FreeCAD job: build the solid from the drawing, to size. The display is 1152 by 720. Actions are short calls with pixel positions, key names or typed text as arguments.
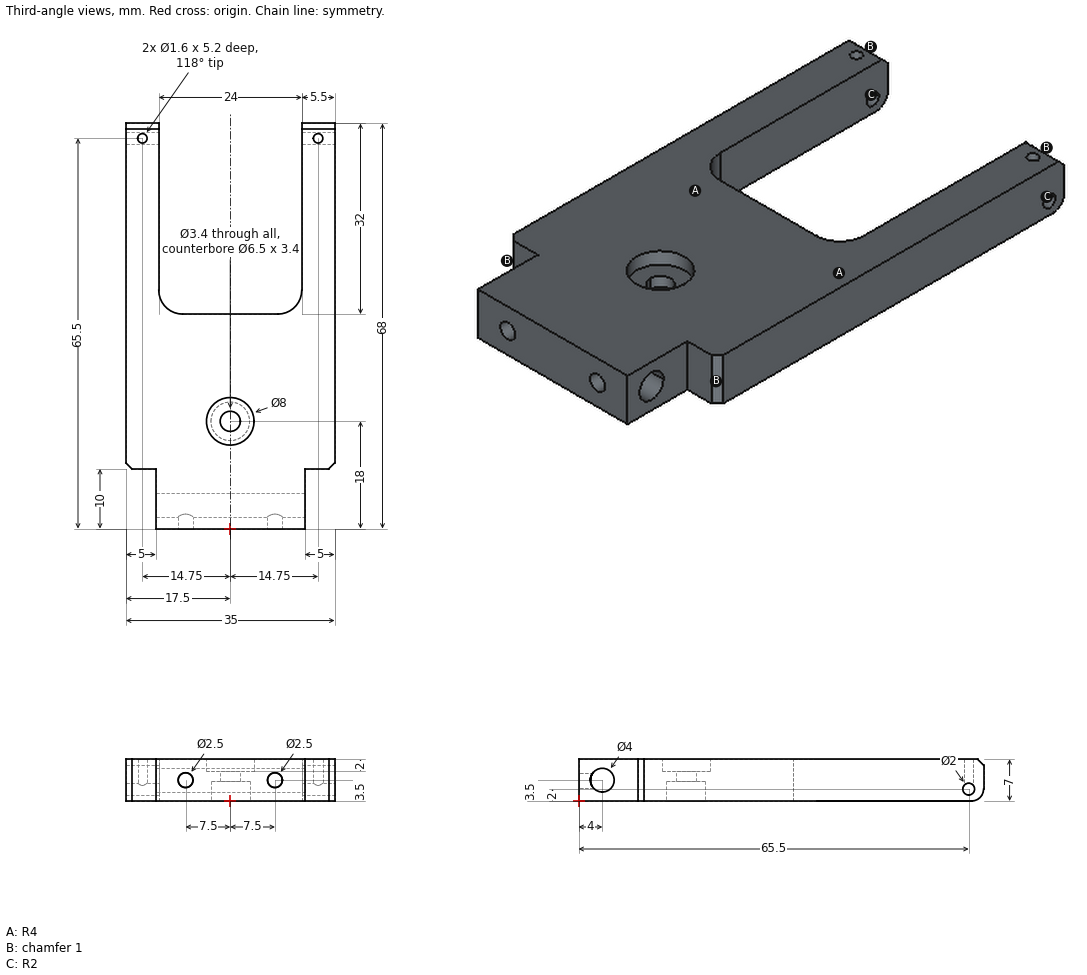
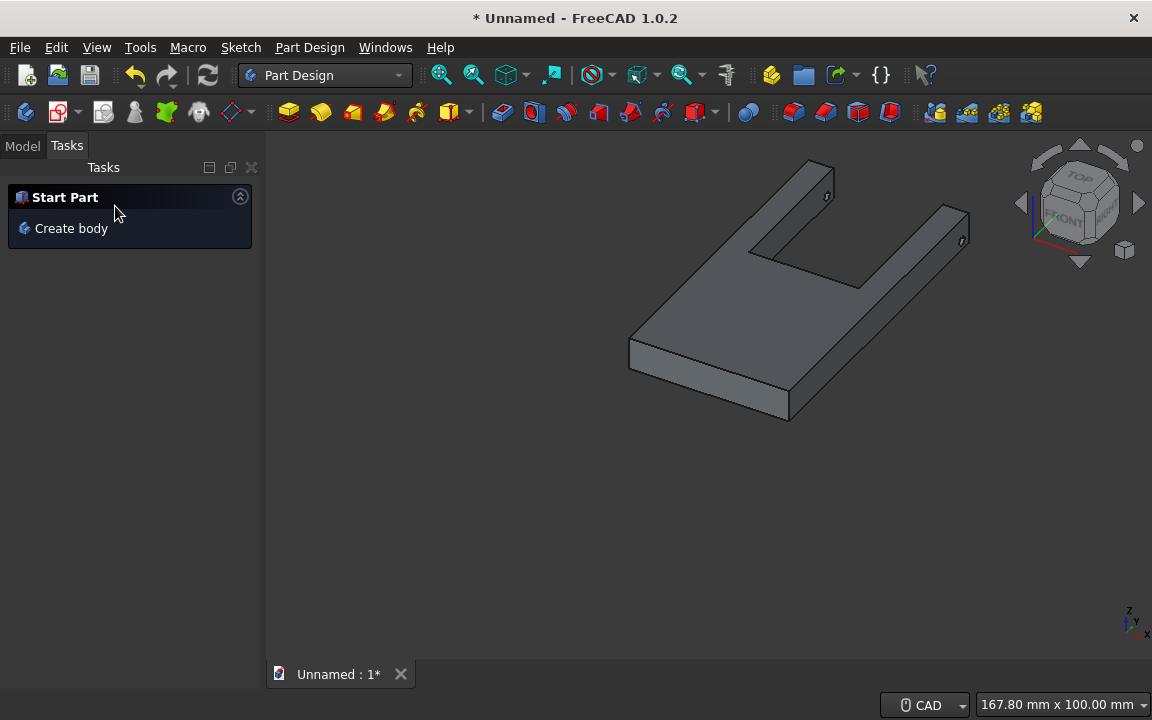
click(747, 326)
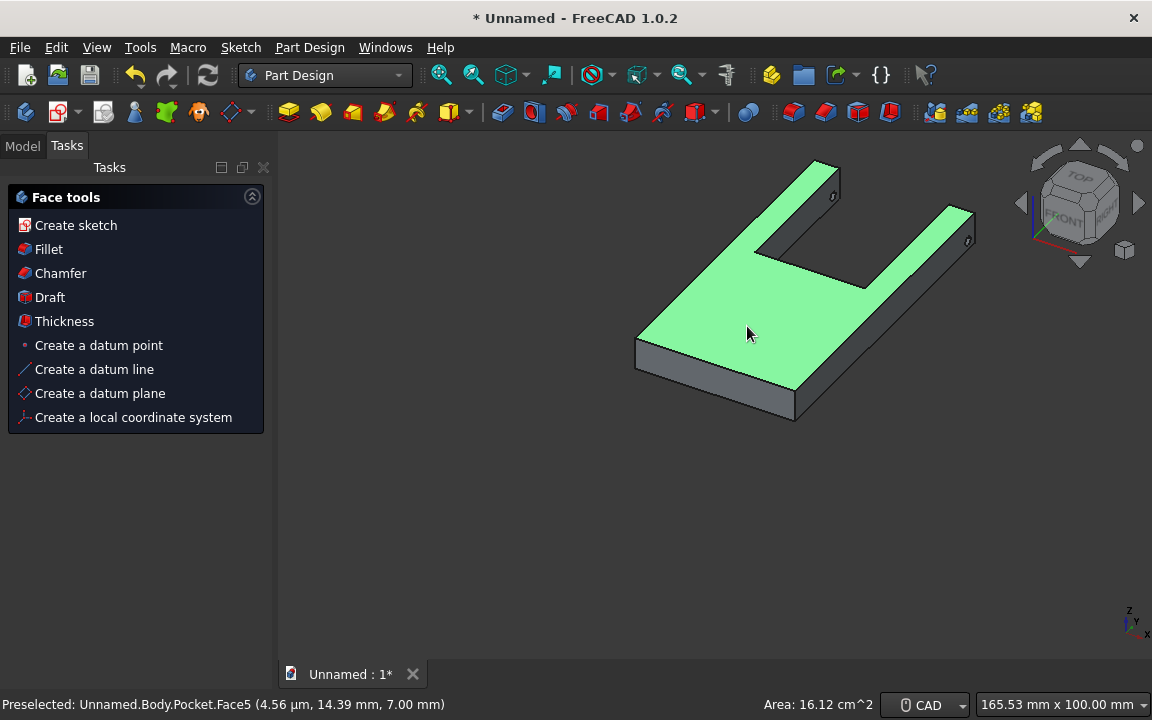
click(58, 112)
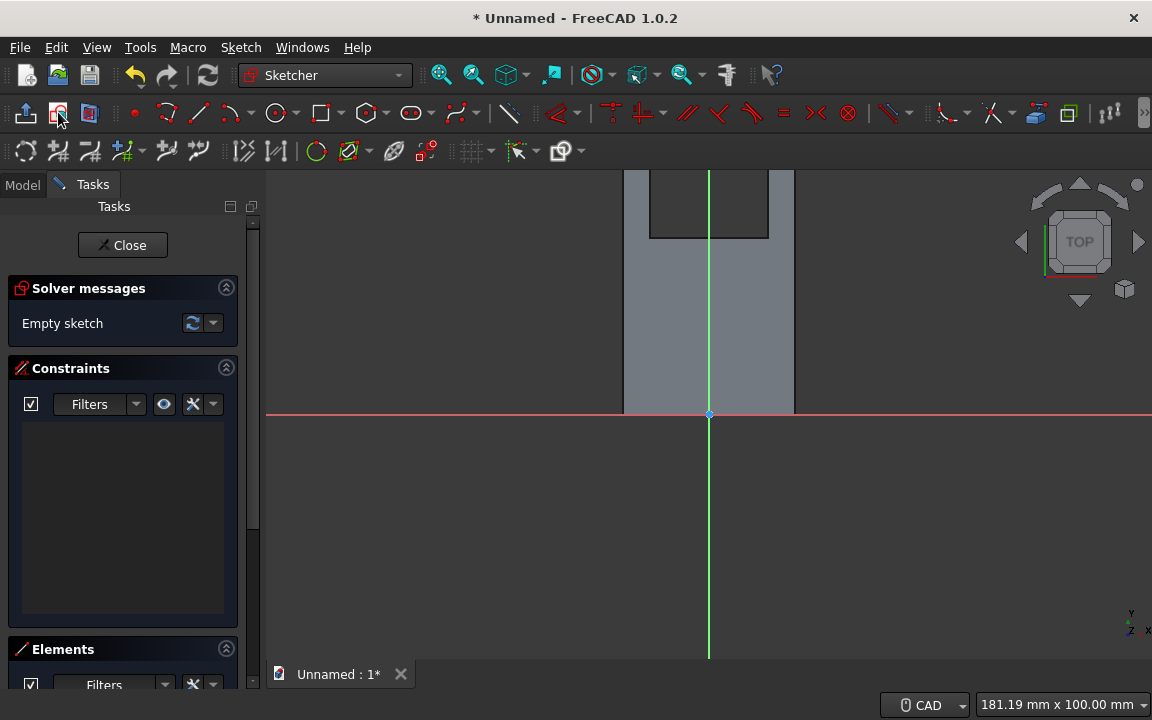
scroll(749, 376, up, 5)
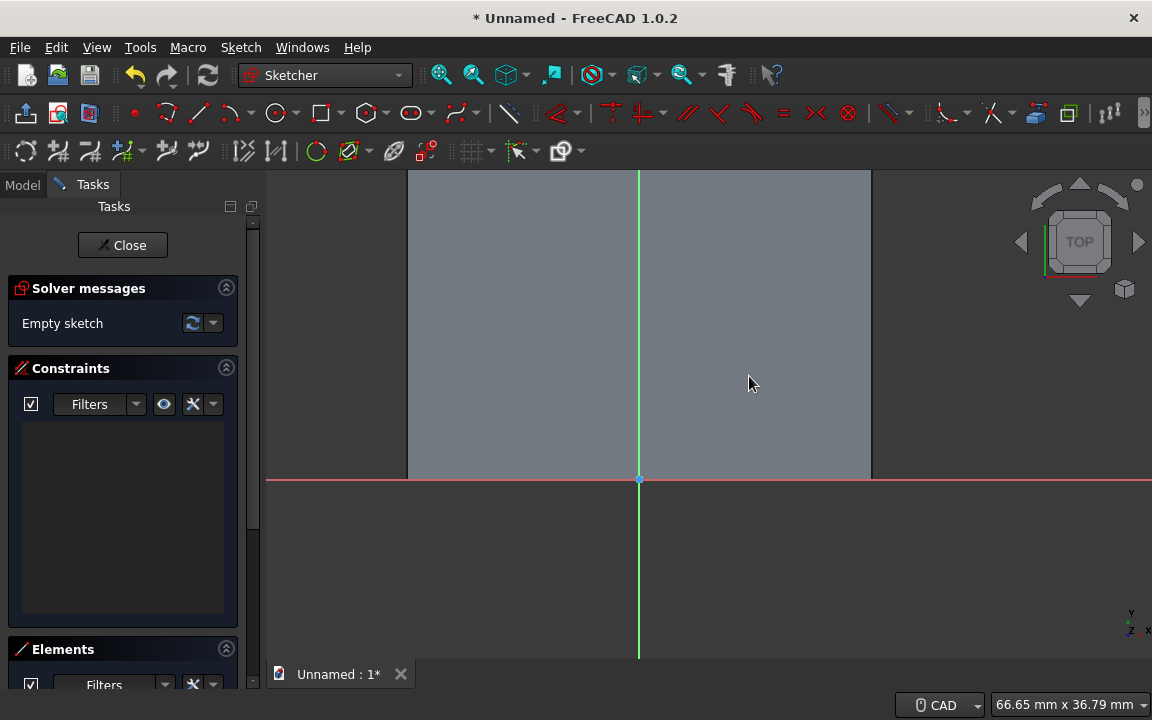
key(g)
key(r)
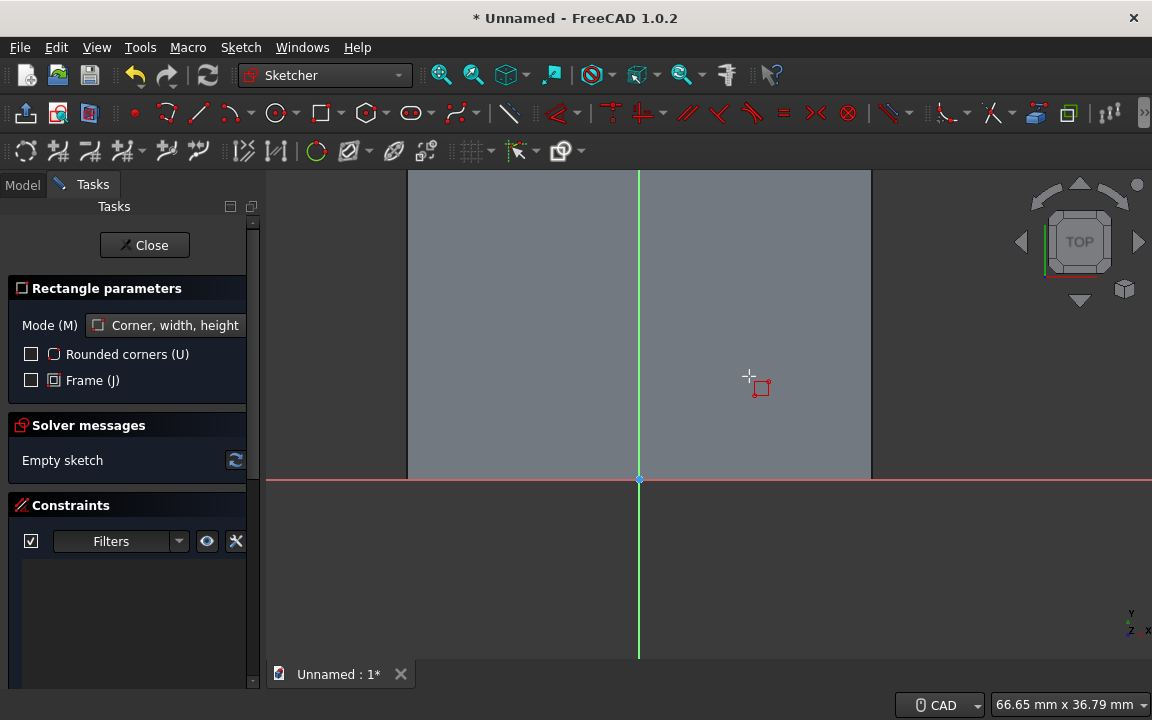
click(407, 347)
click(473, 480)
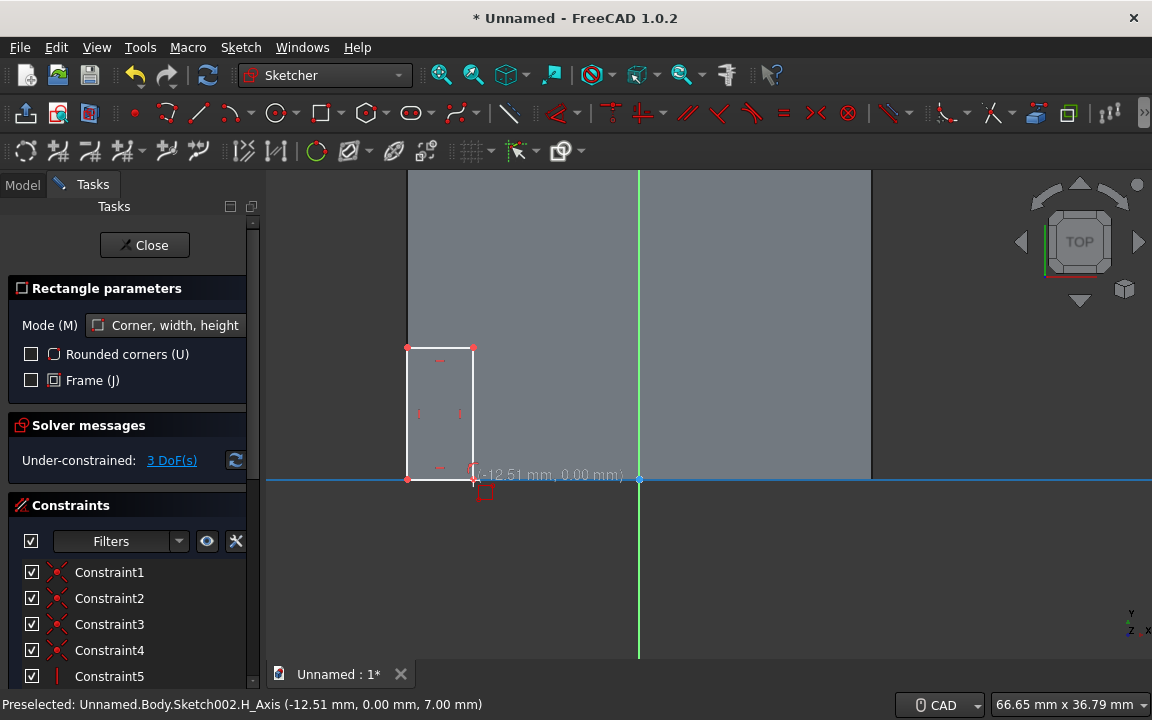
click(805, 347)
click(872, 480)
key(Escape)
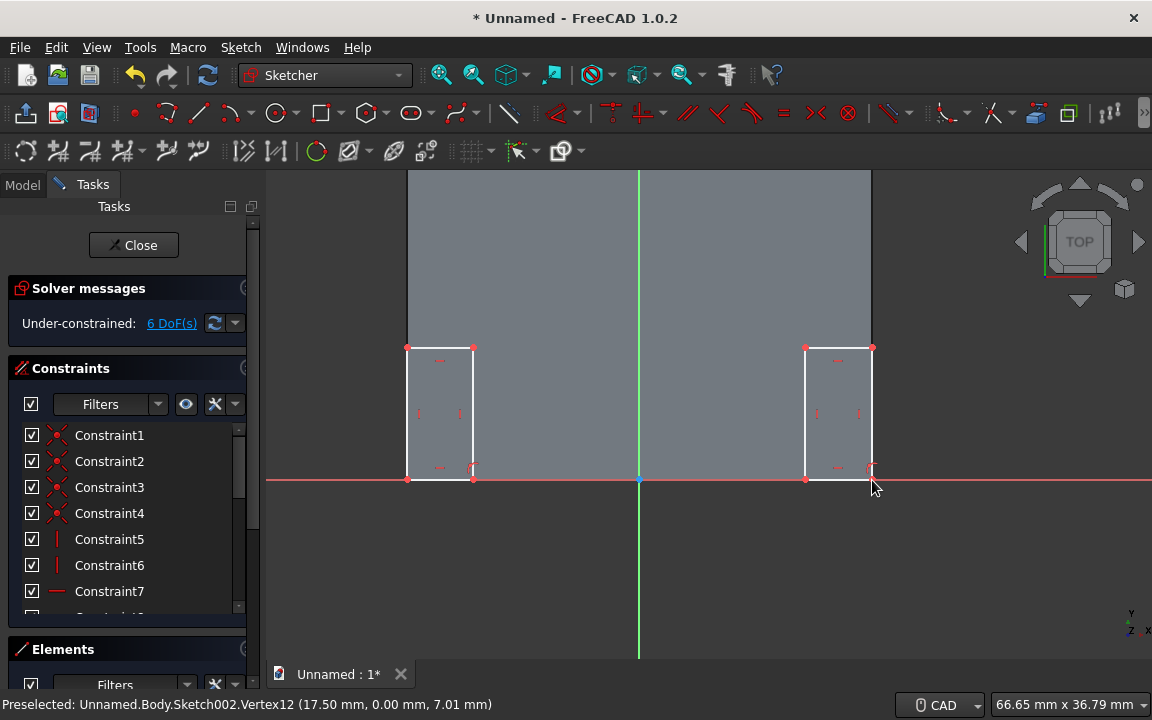
click(473, 348)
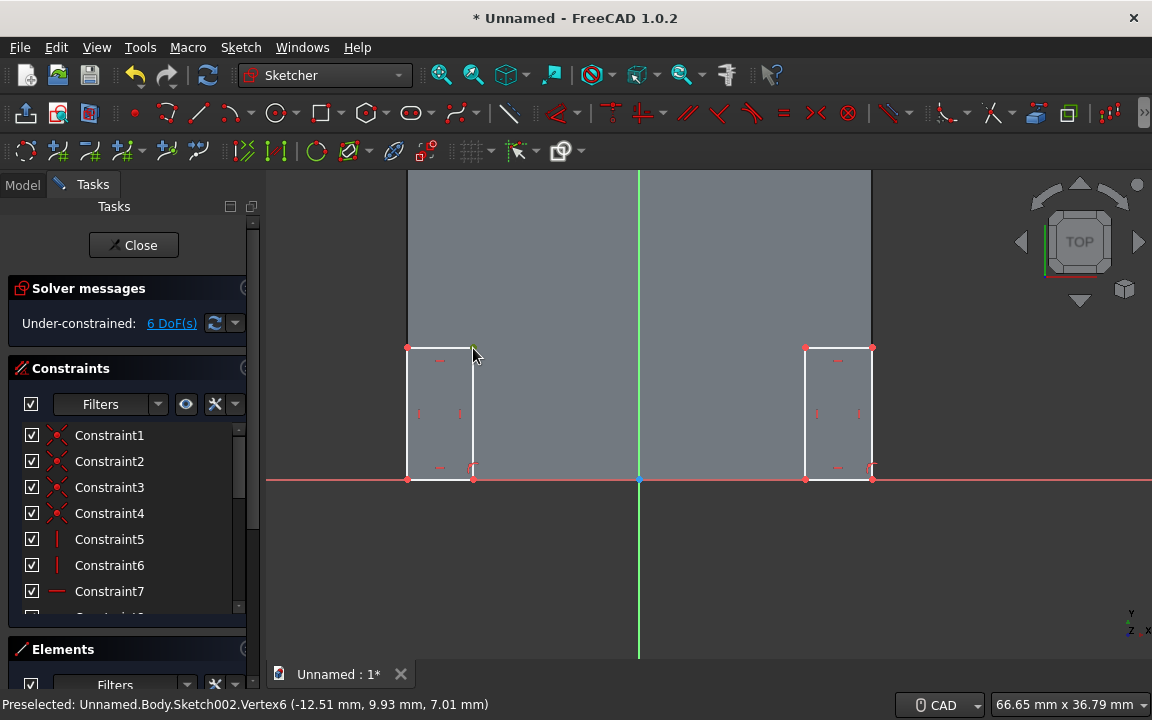
click(805, 348)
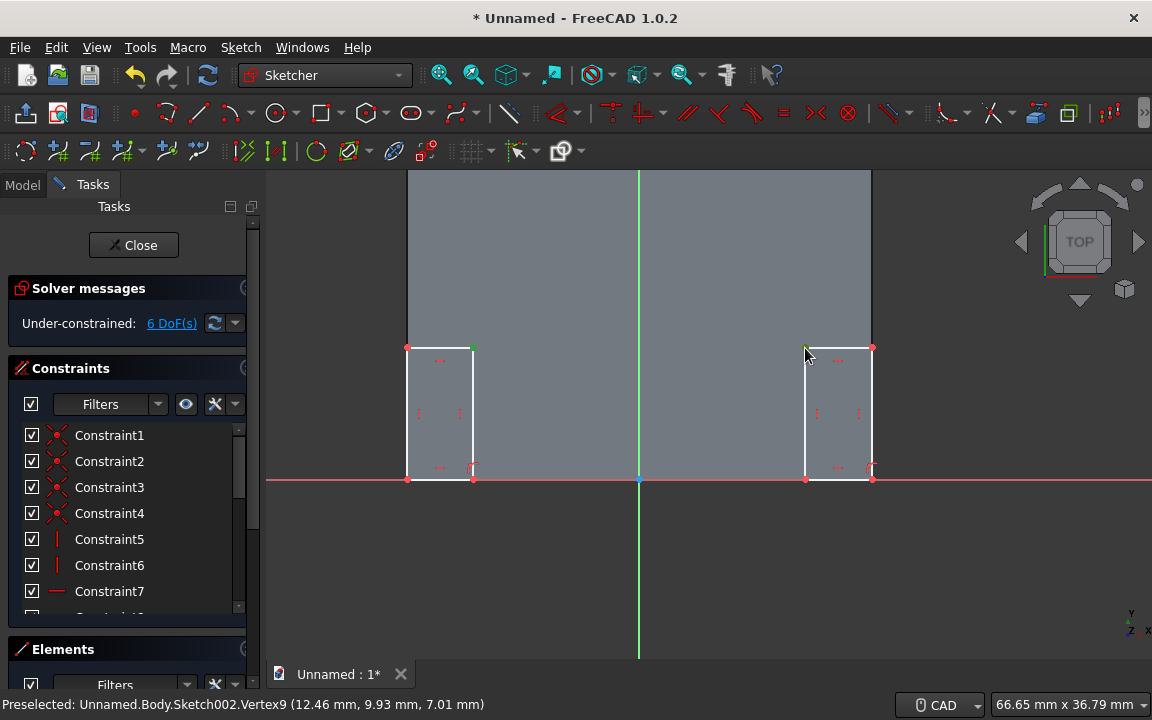
click(639, 600)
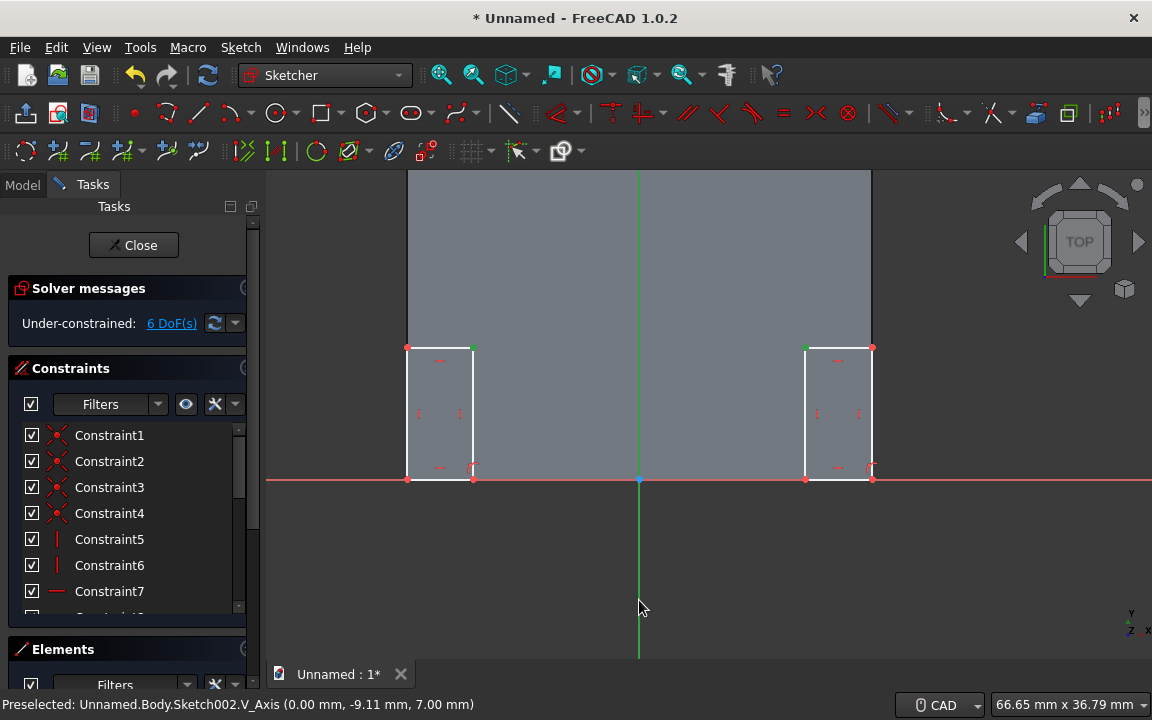
key(s)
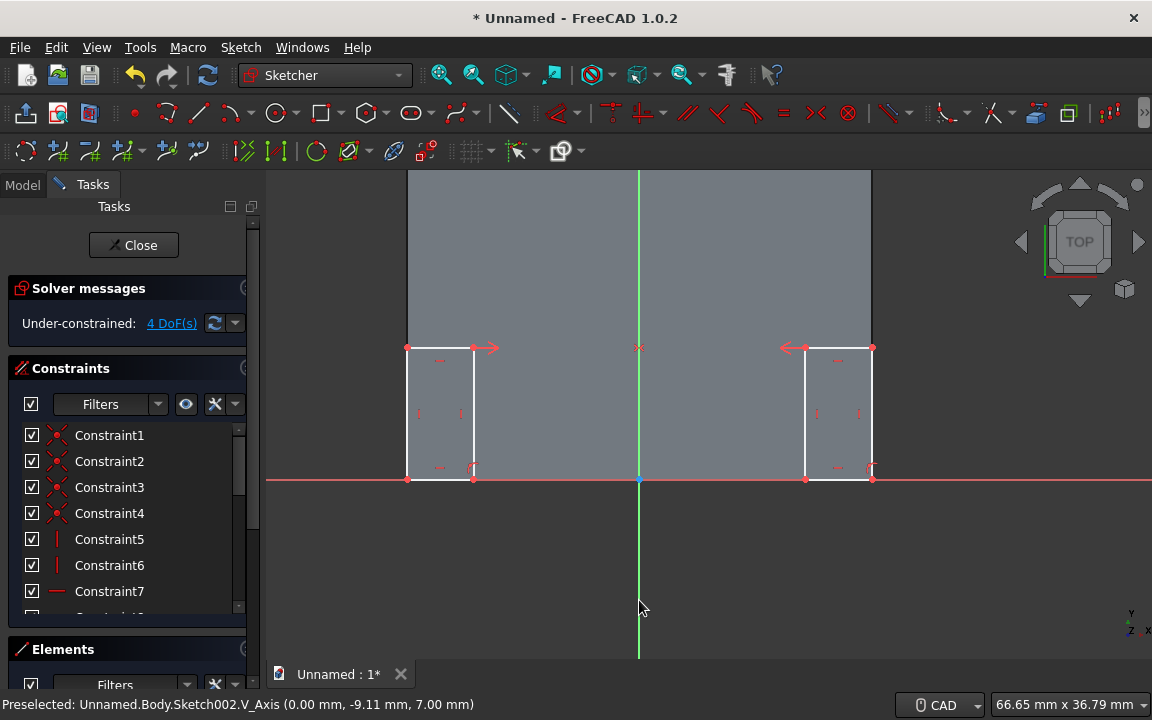
key(d)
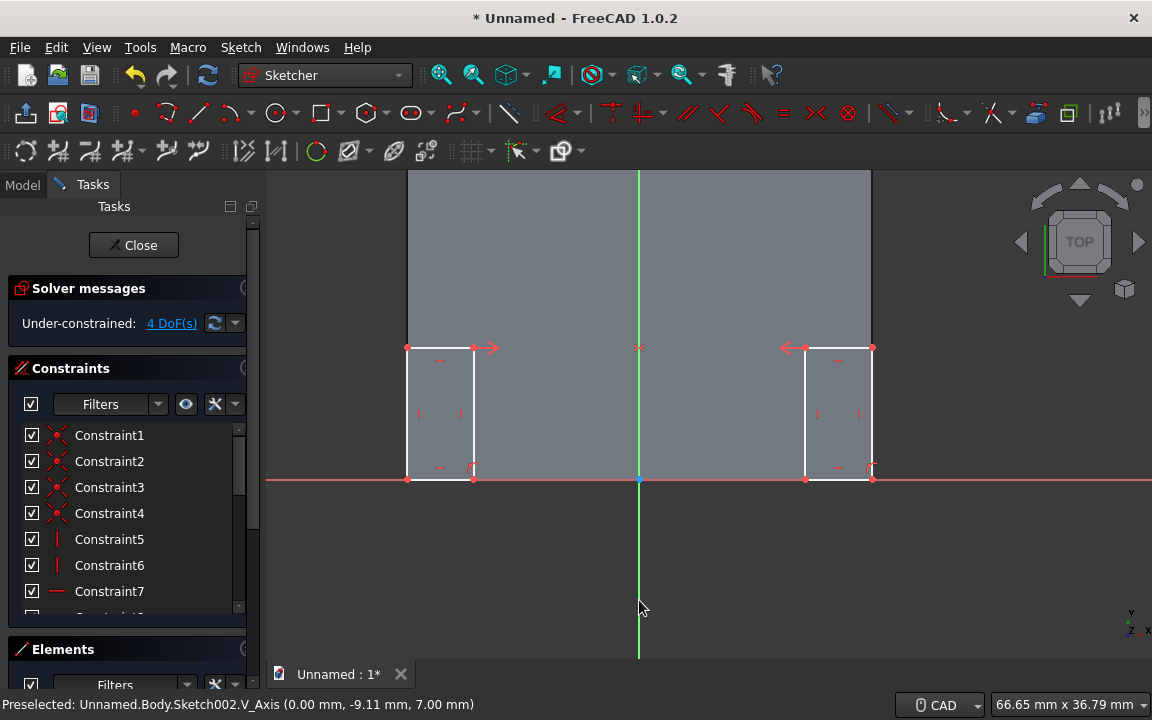
click(427, 480)
click(440, 514)